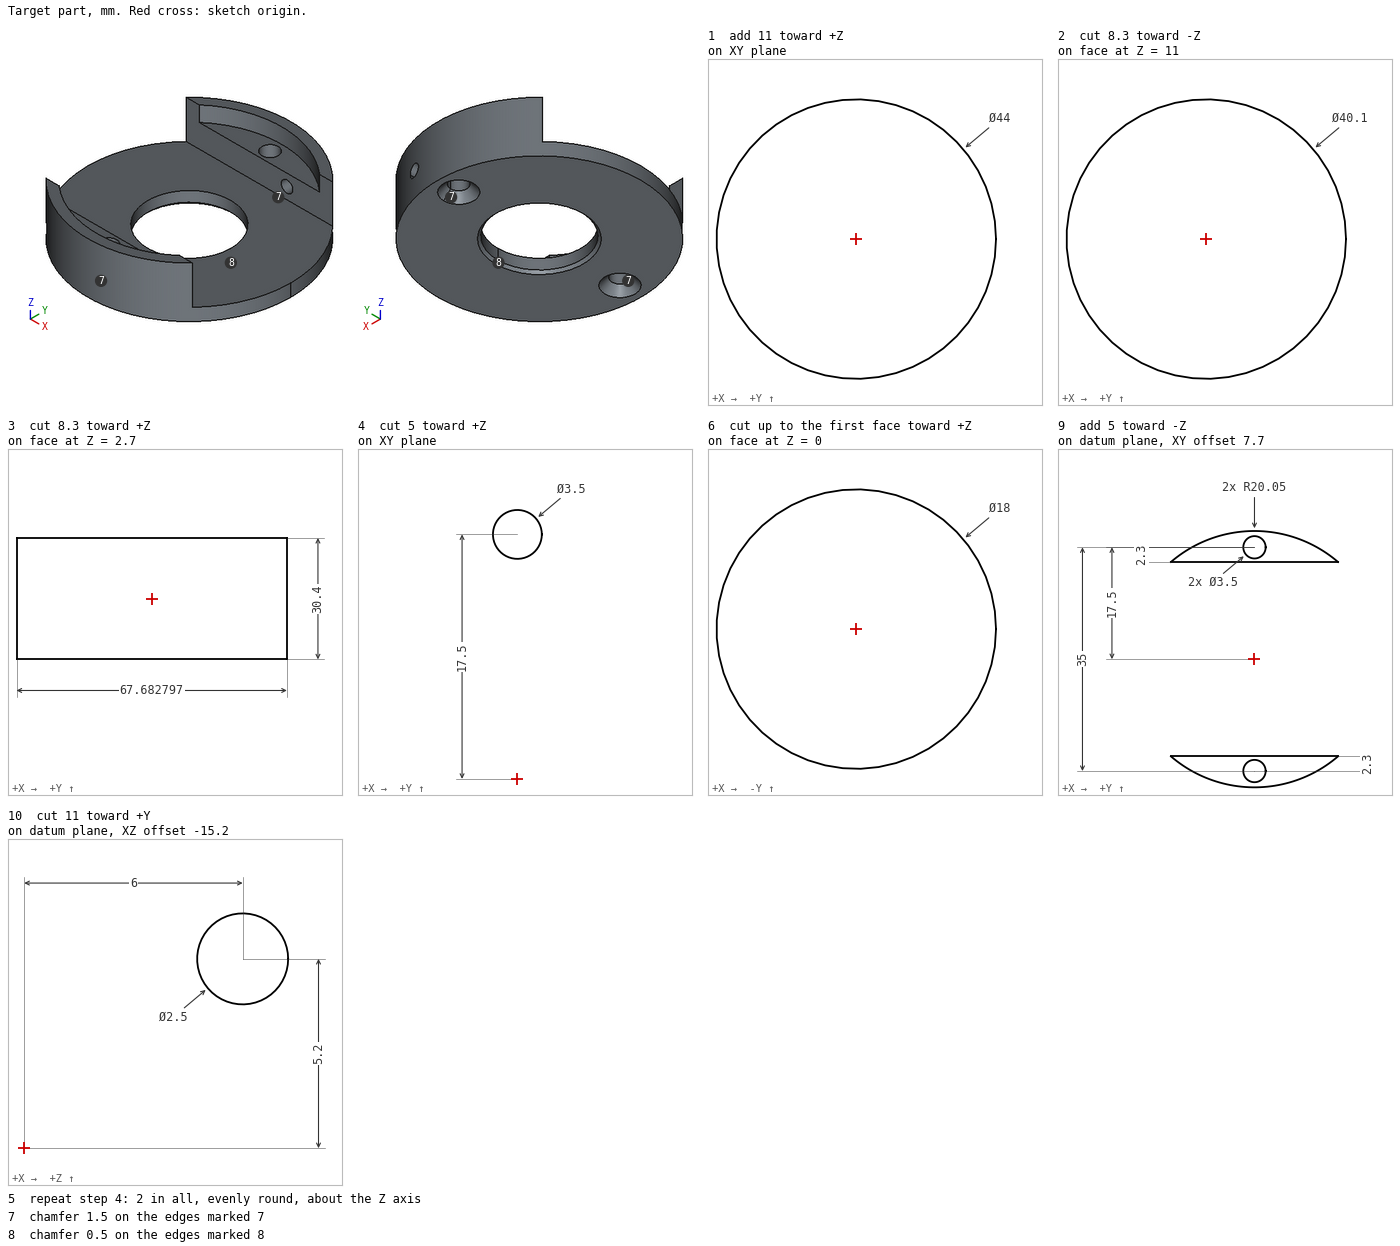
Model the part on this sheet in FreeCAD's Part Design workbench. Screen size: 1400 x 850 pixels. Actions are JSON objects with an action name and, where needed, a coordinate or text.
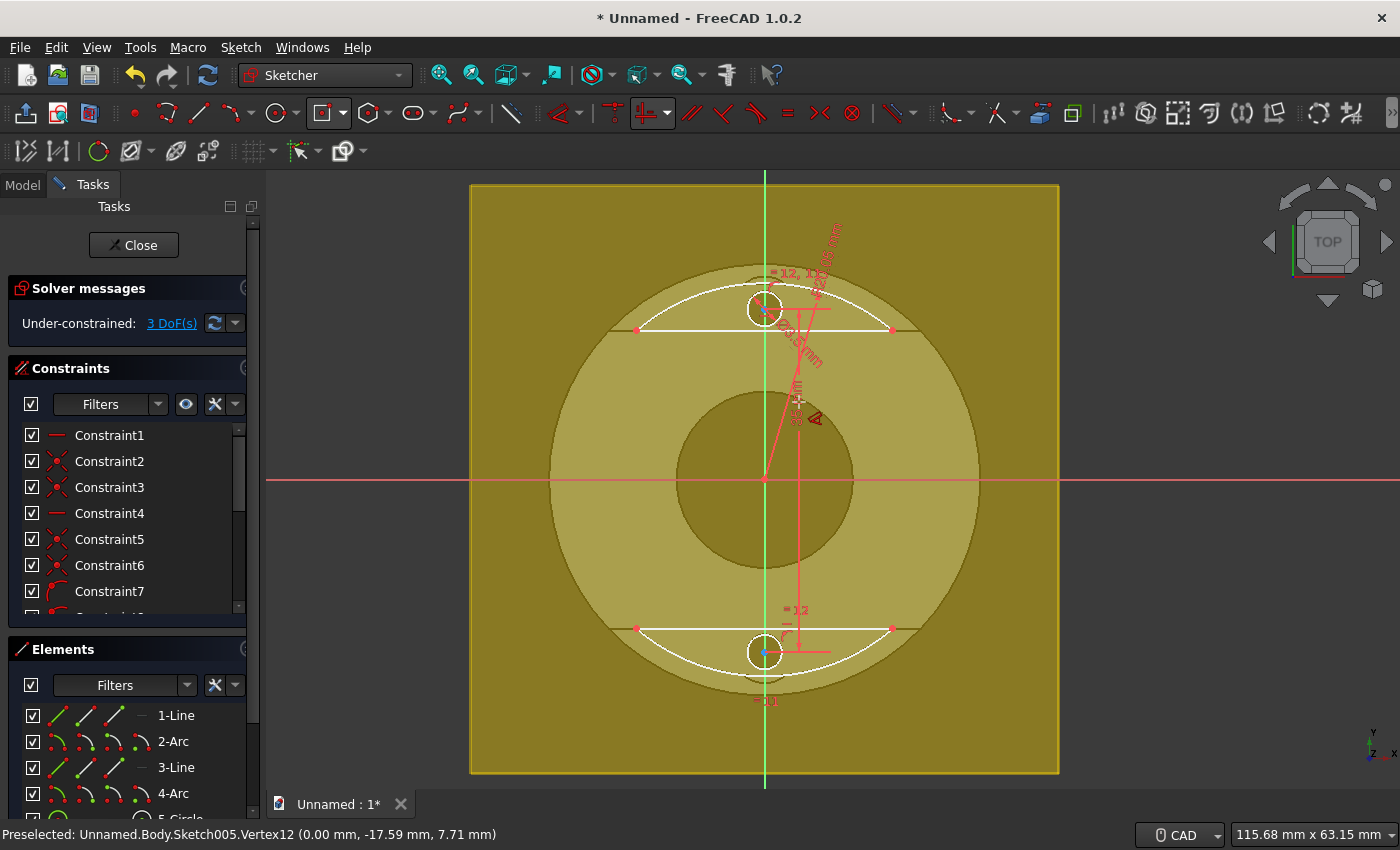
{"action": "left_click", "coordinate": [765, 309]}
{"action": "left_click", "coordinate": [799, 434]}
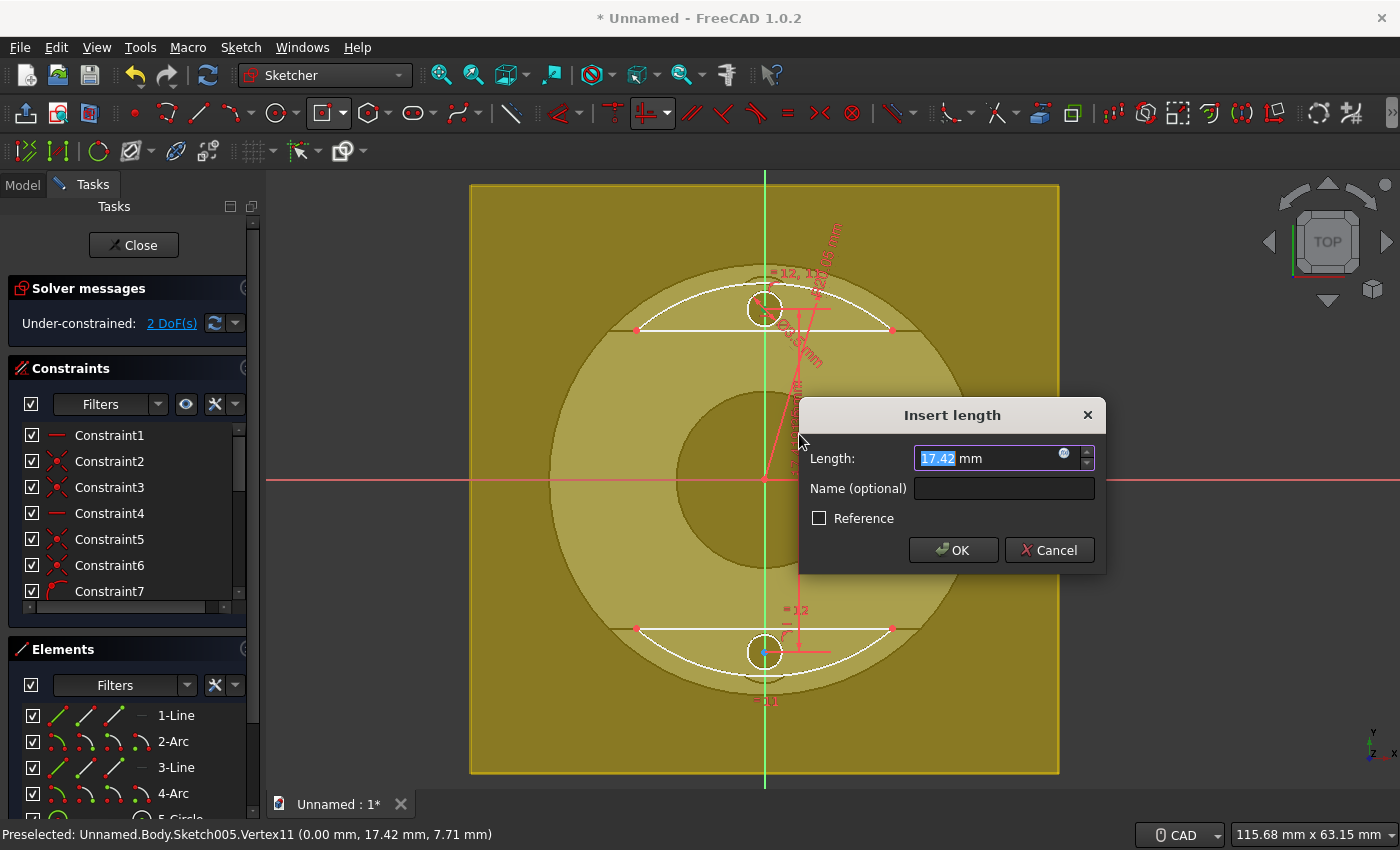
{"action": "type", "text": "17.5"}
{"action": "key", "text": "Return"}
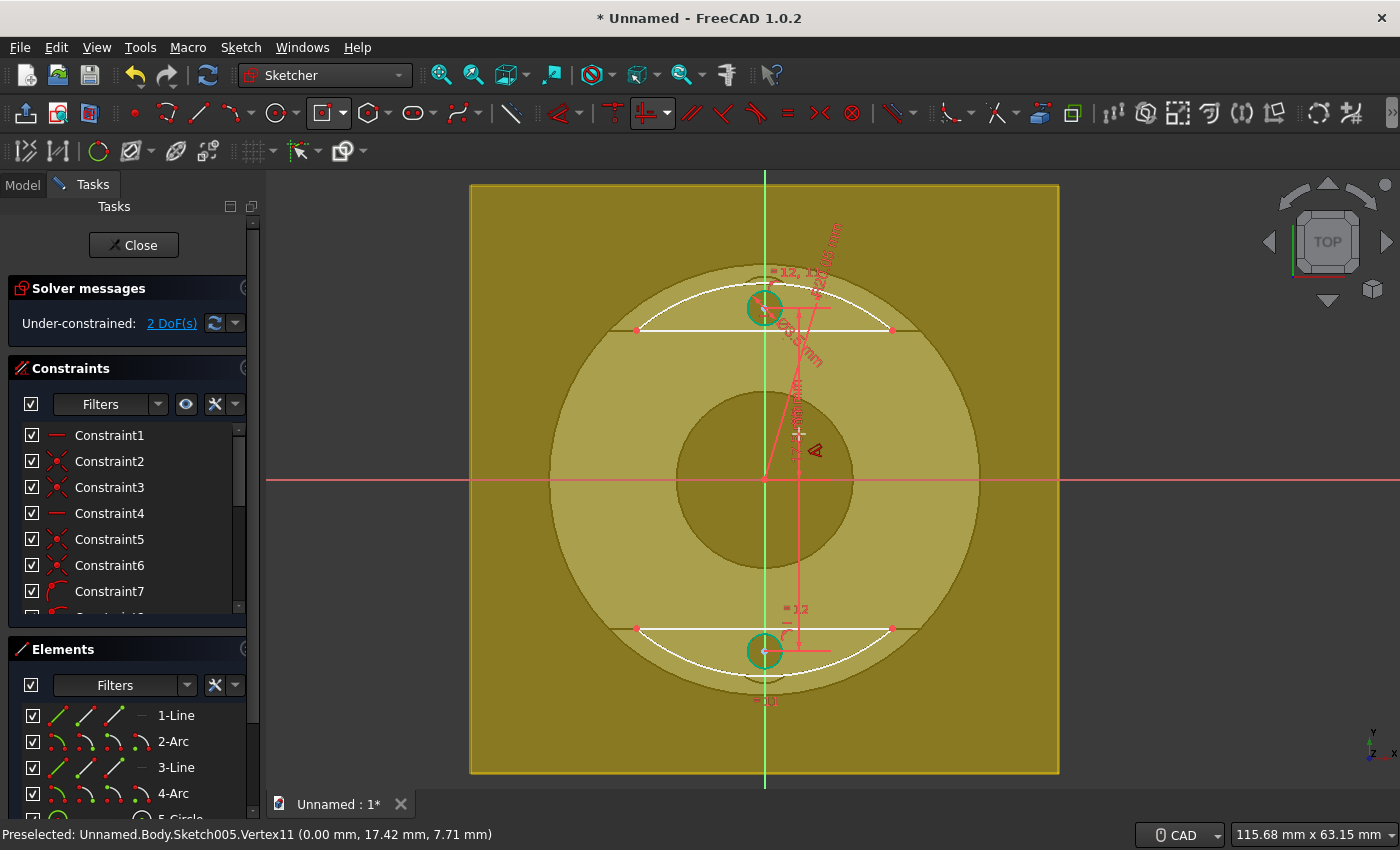
{"action": "scroll", "coordinate": [637, 331], "scroll_direction": "up", "scroll_amount": 3}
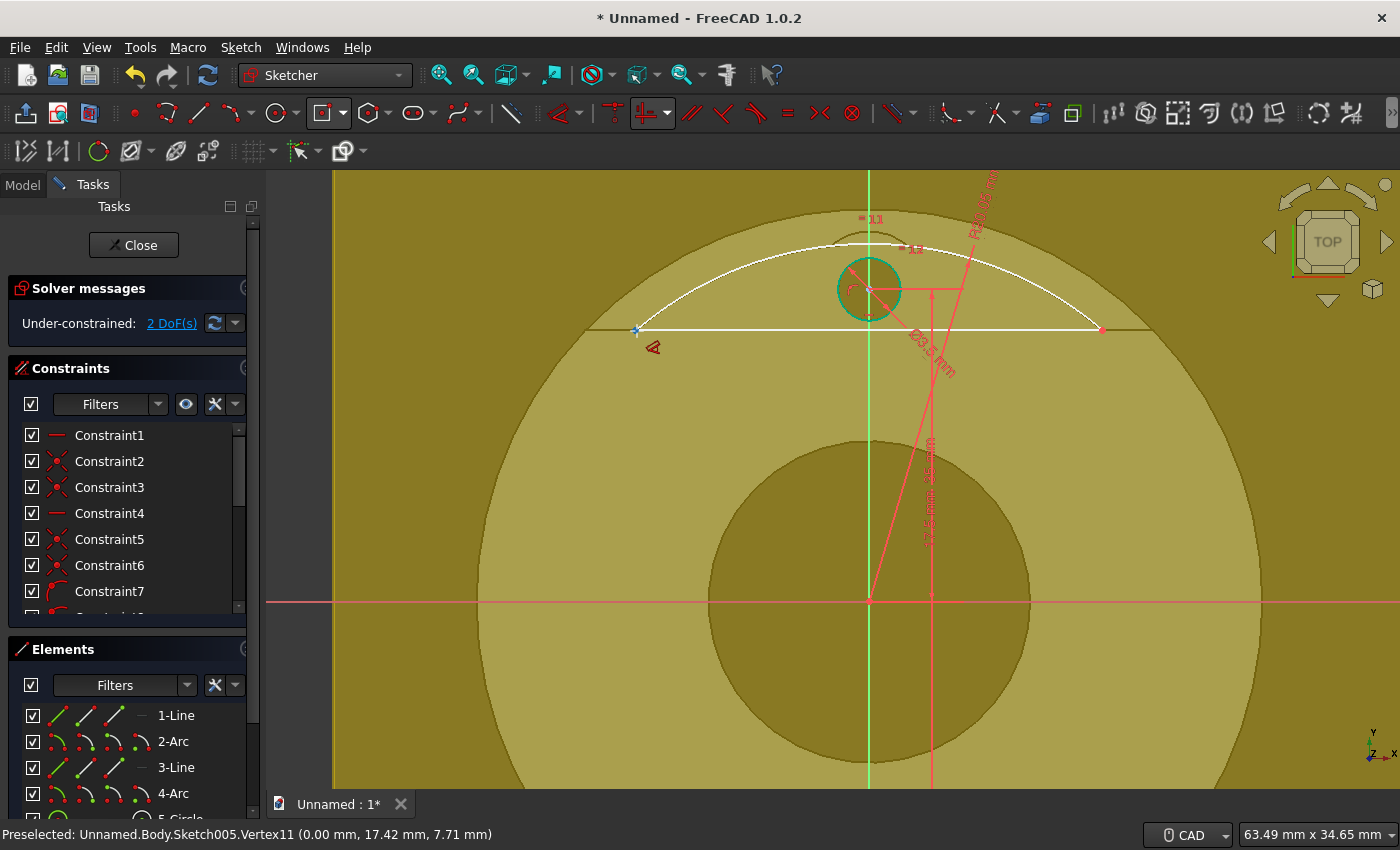
{"action": "left_click", "coordinate": [636, 330]}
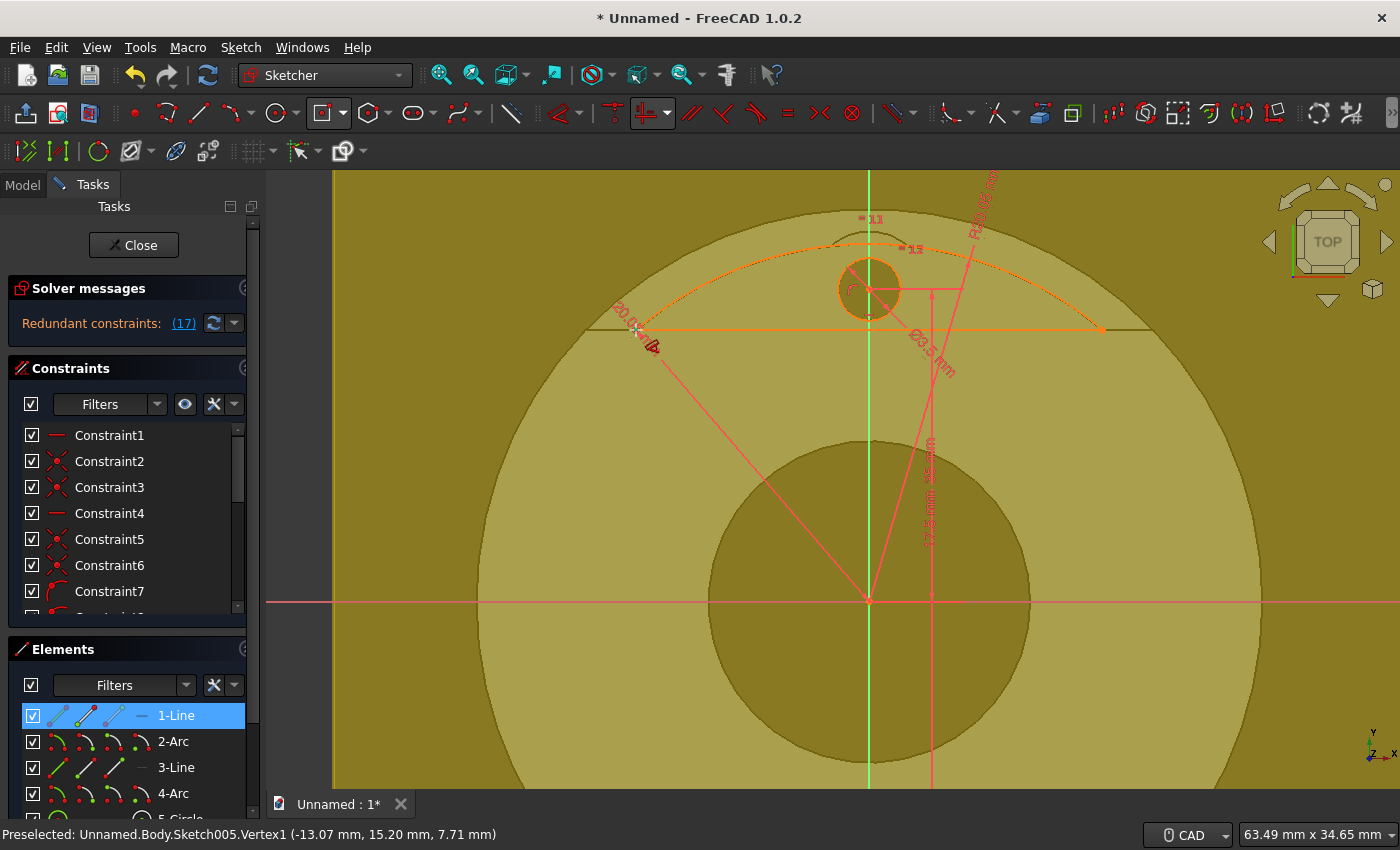
{"action": "left_click", "coordinate": [869, 289]}
{"action": "left_click", "coordinate": [602, 310]}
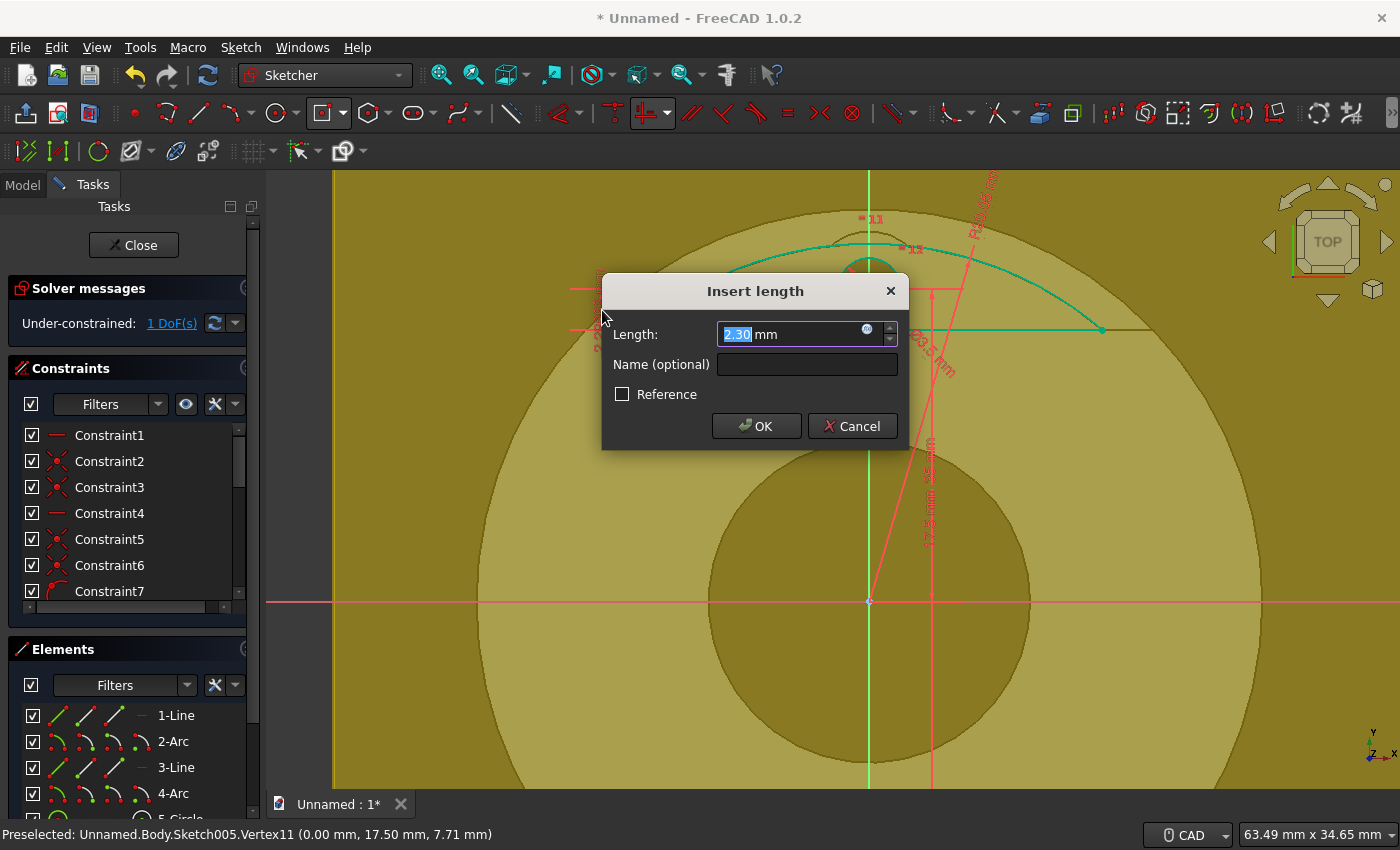
{"action": "type", "text": "2.3"}
{"action": "key", "text": "Return"}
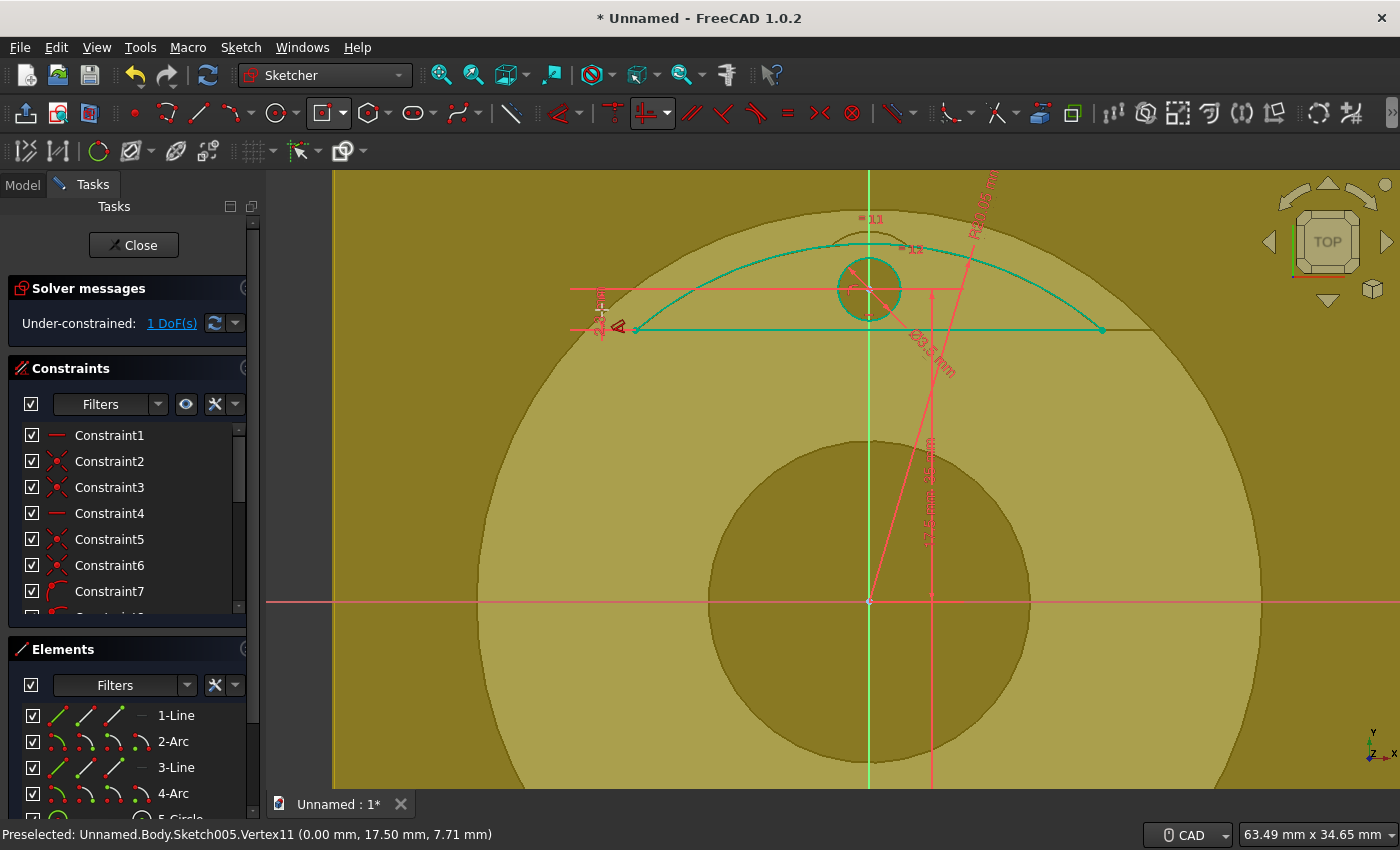
{"action": "scroll", "coordinate": [637, 331], "scroll_direction": "down", "scroll_amount": 3}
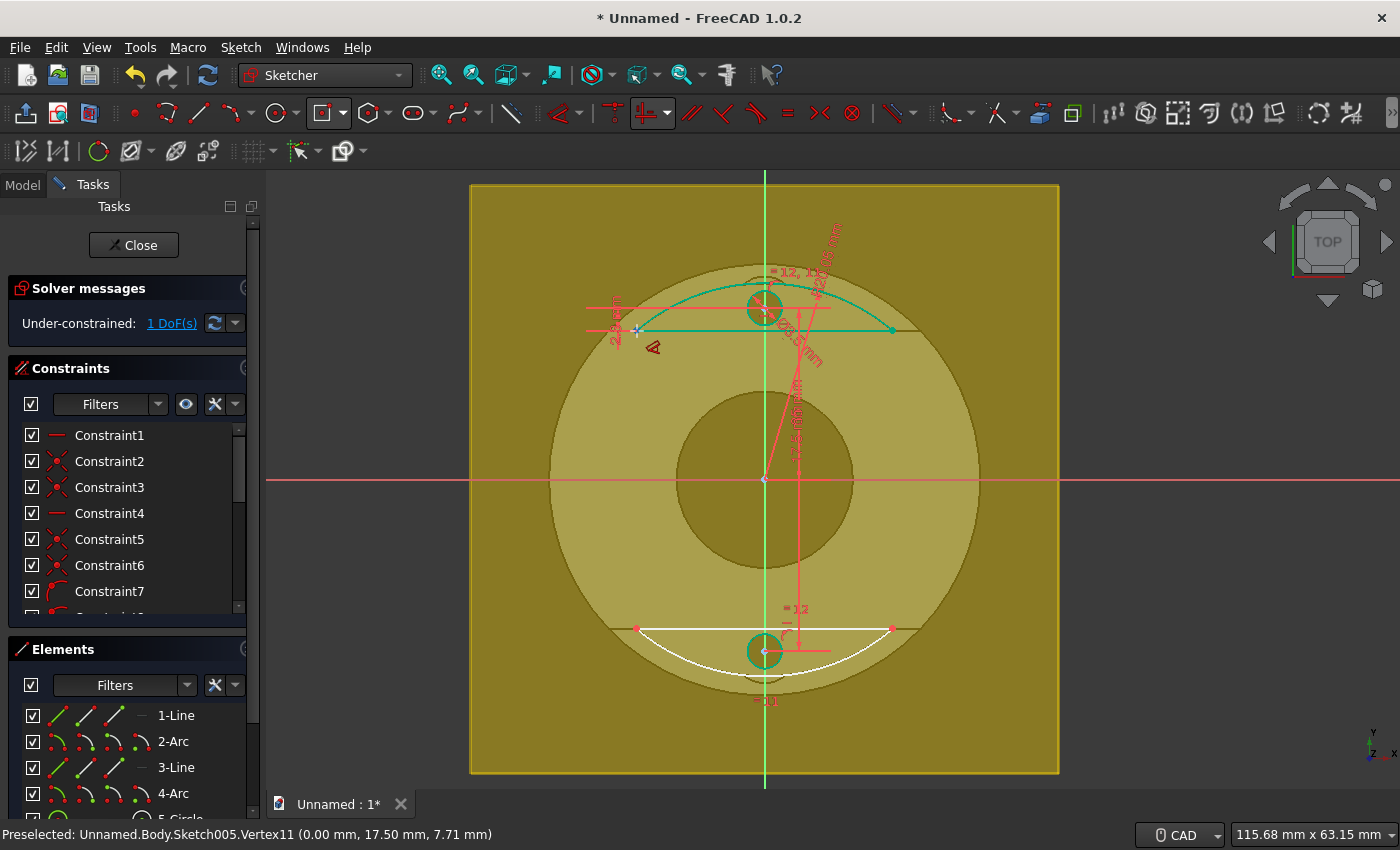
{"action": "scroll", "coordinate": [893, 629], "scroll_direction": "up", "scroll_amount": 3}